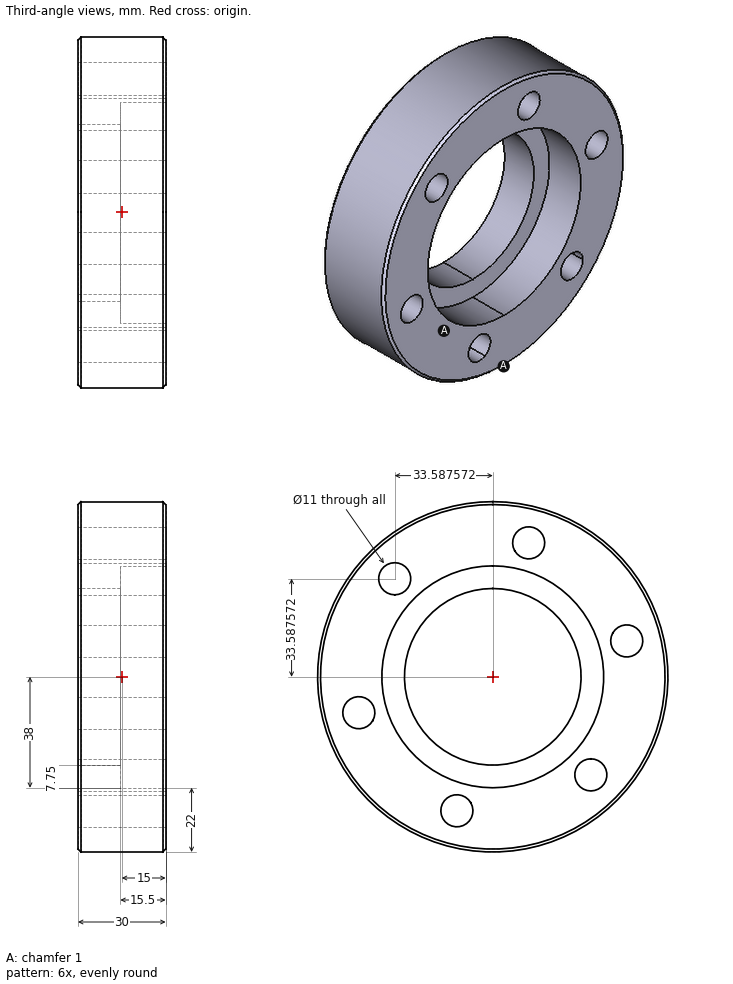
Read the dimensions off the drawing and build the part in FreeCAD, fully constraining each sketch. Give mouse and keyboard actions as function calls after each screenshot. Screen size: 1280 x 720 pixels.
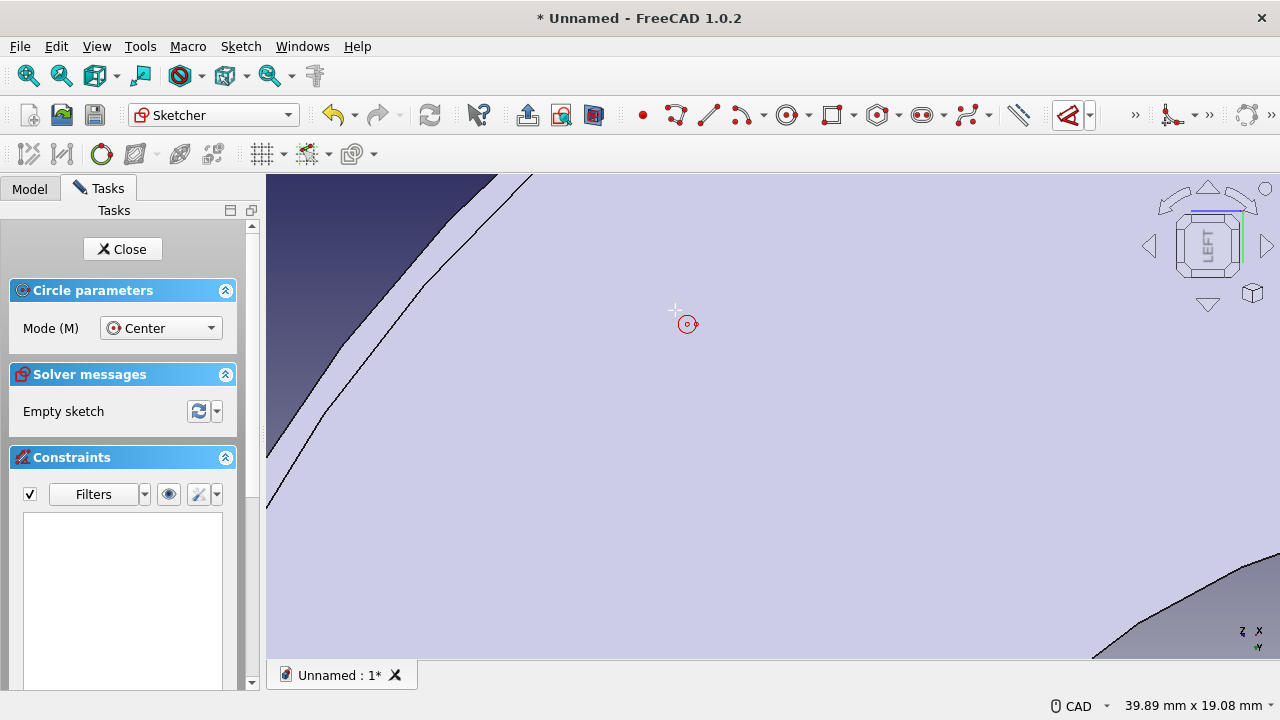
click(703, 415)
move(801, 316)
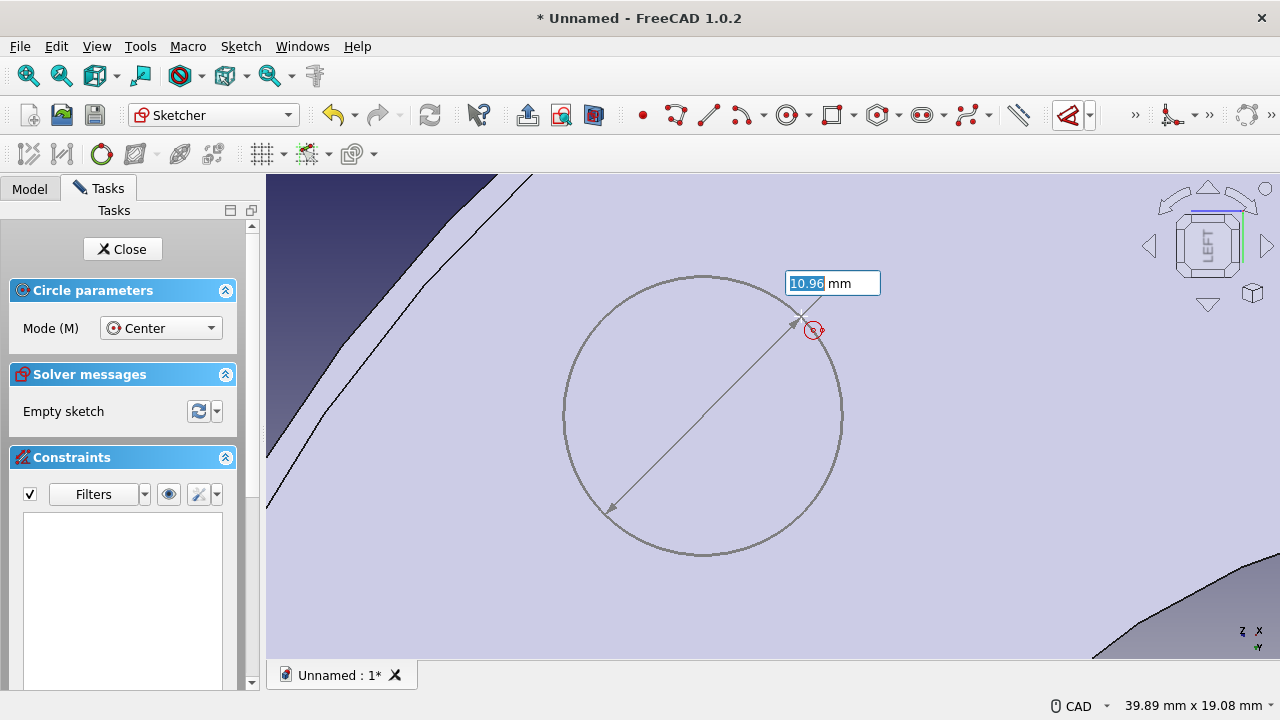
text(11)
key(Return)
key(Escape)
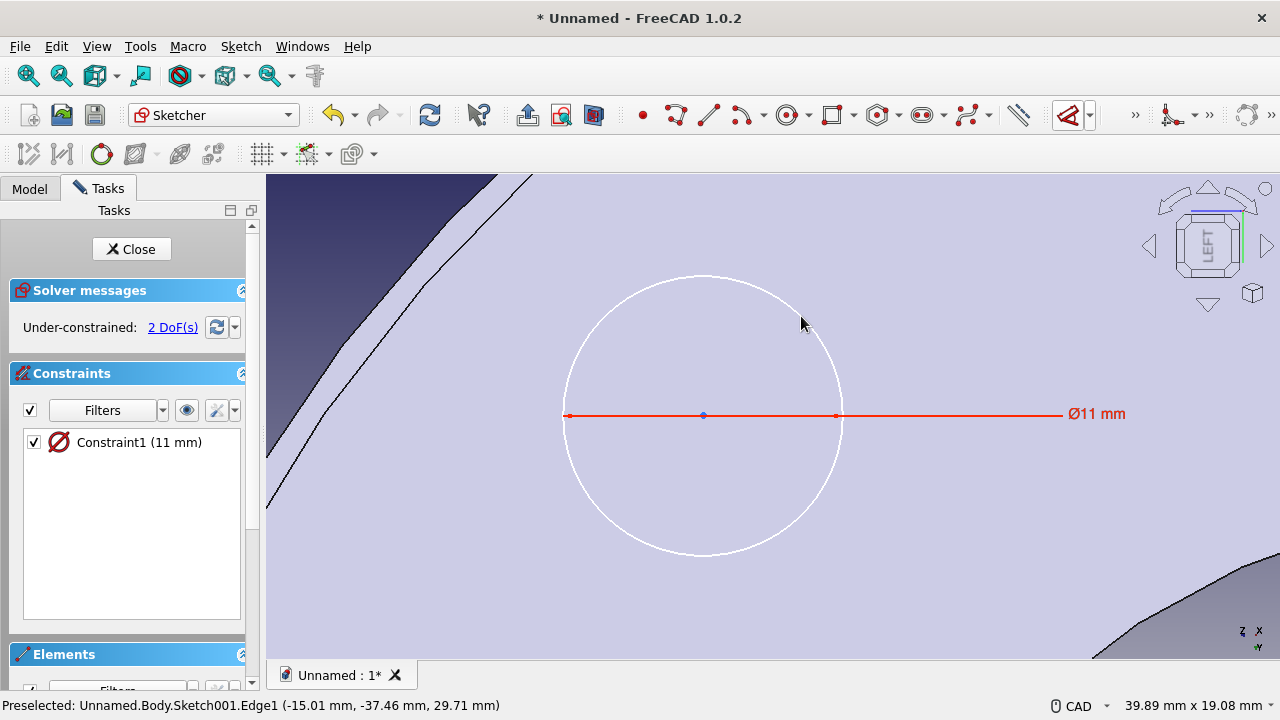
click(703, 416)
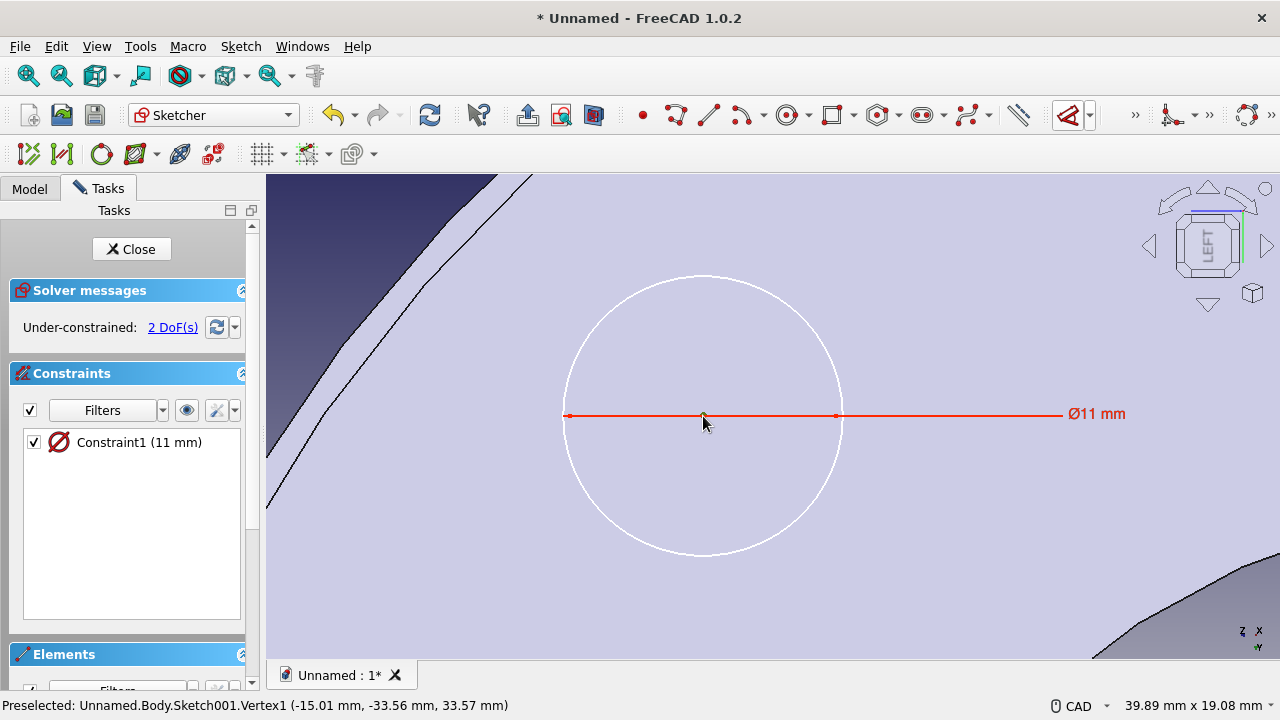
key(l)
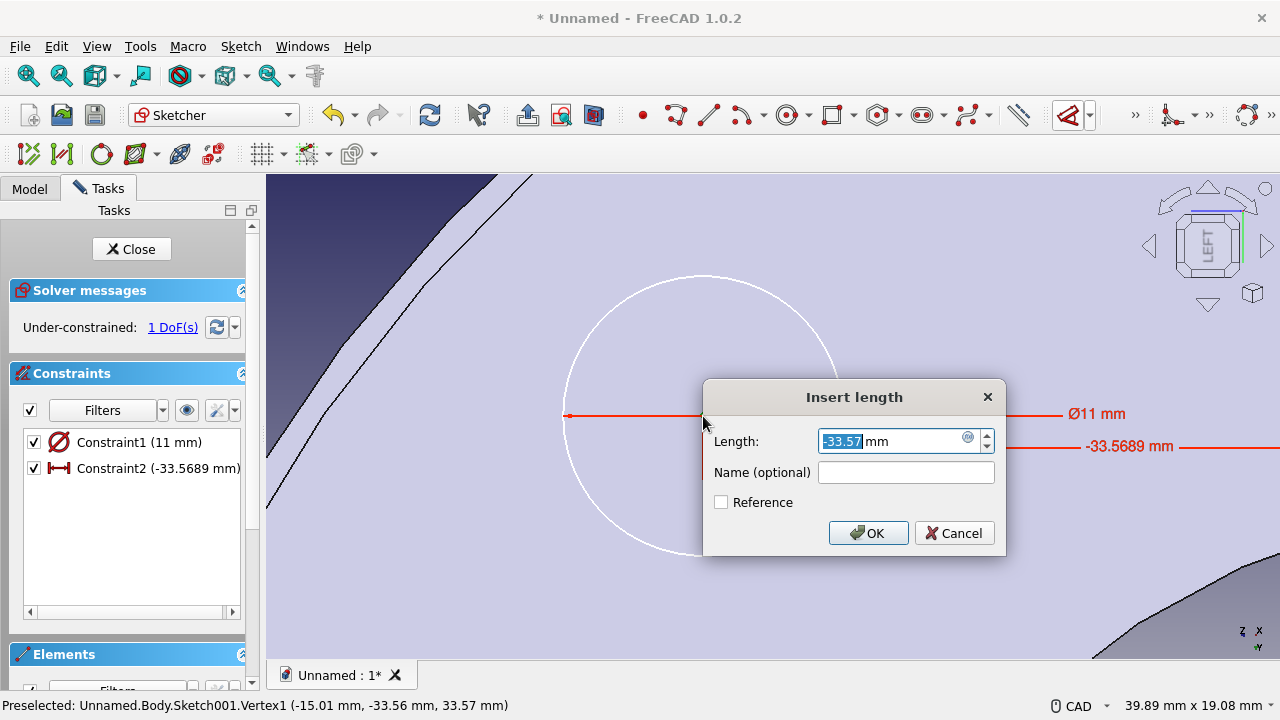
text(-33.587572)
key(Return)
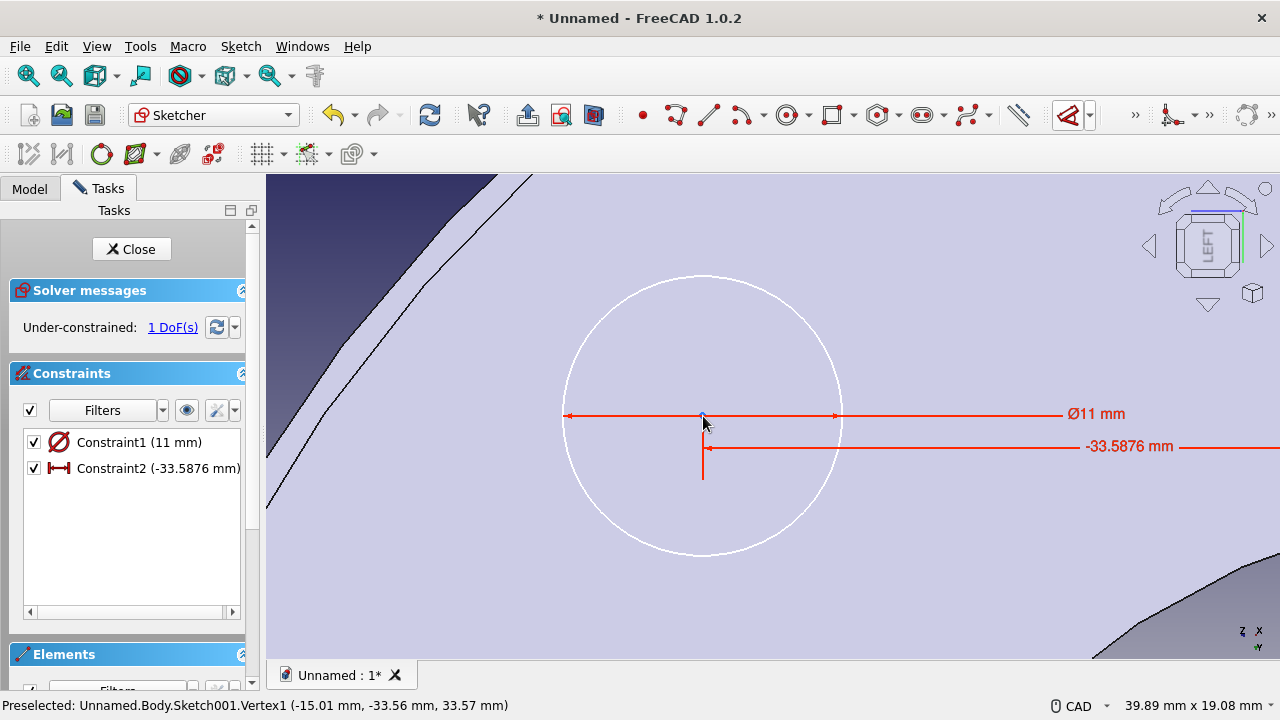
click(703, 416)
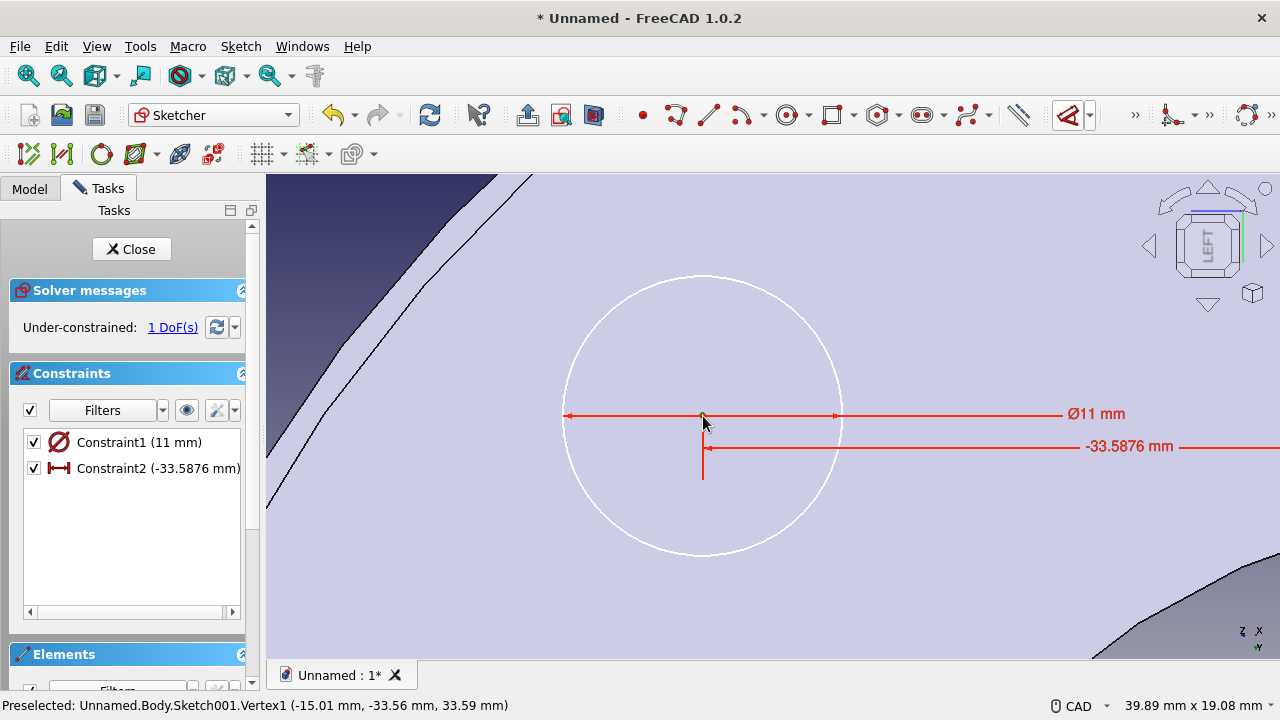
key(i)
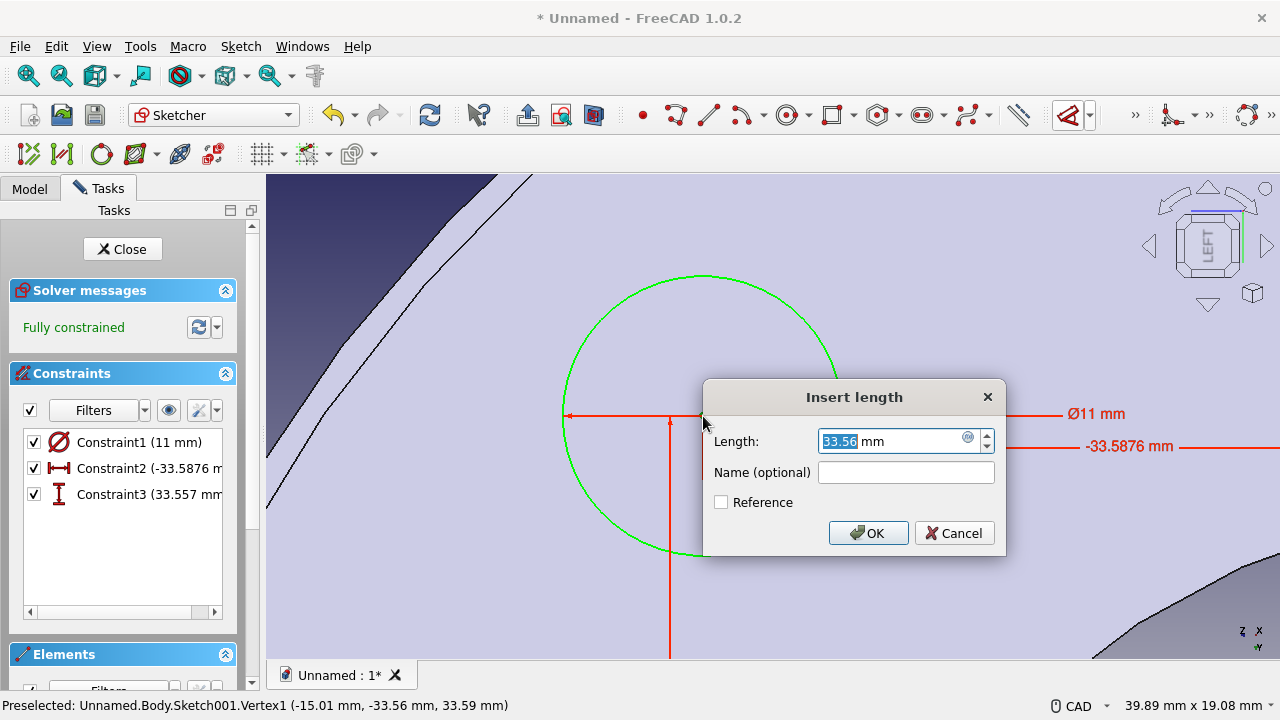
text(33.587572)
key(Return)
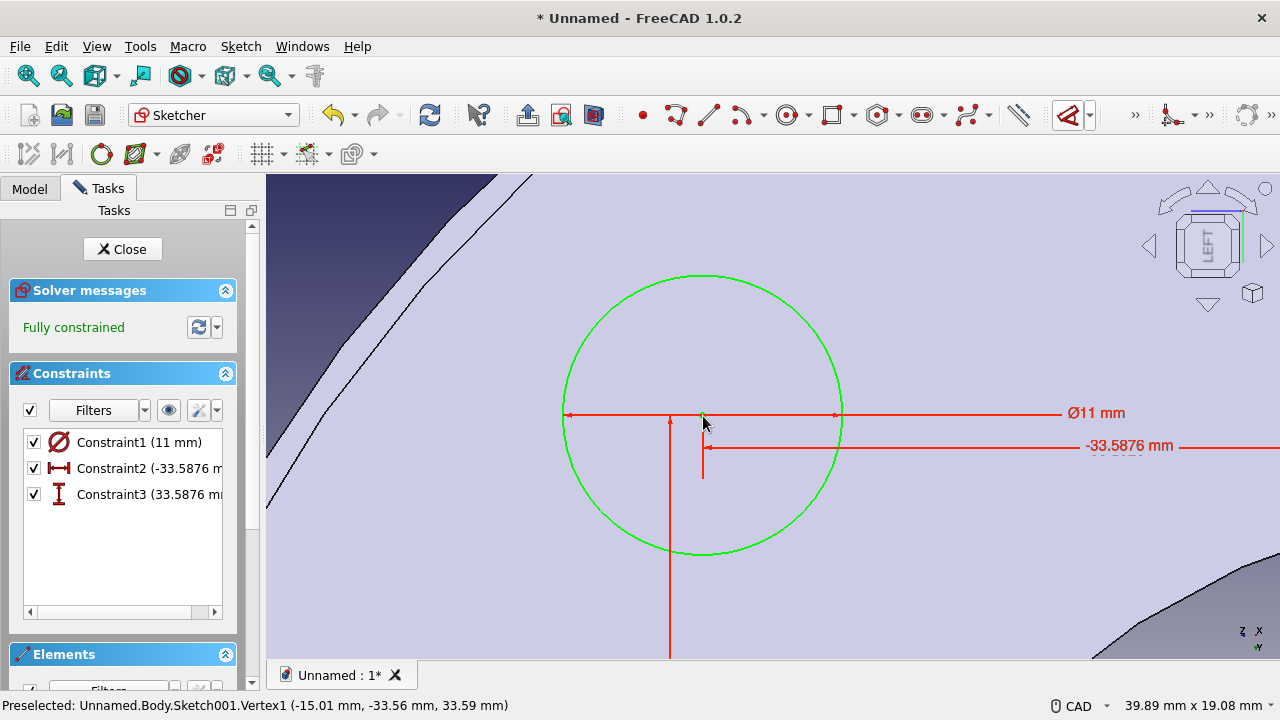
click(123, 249)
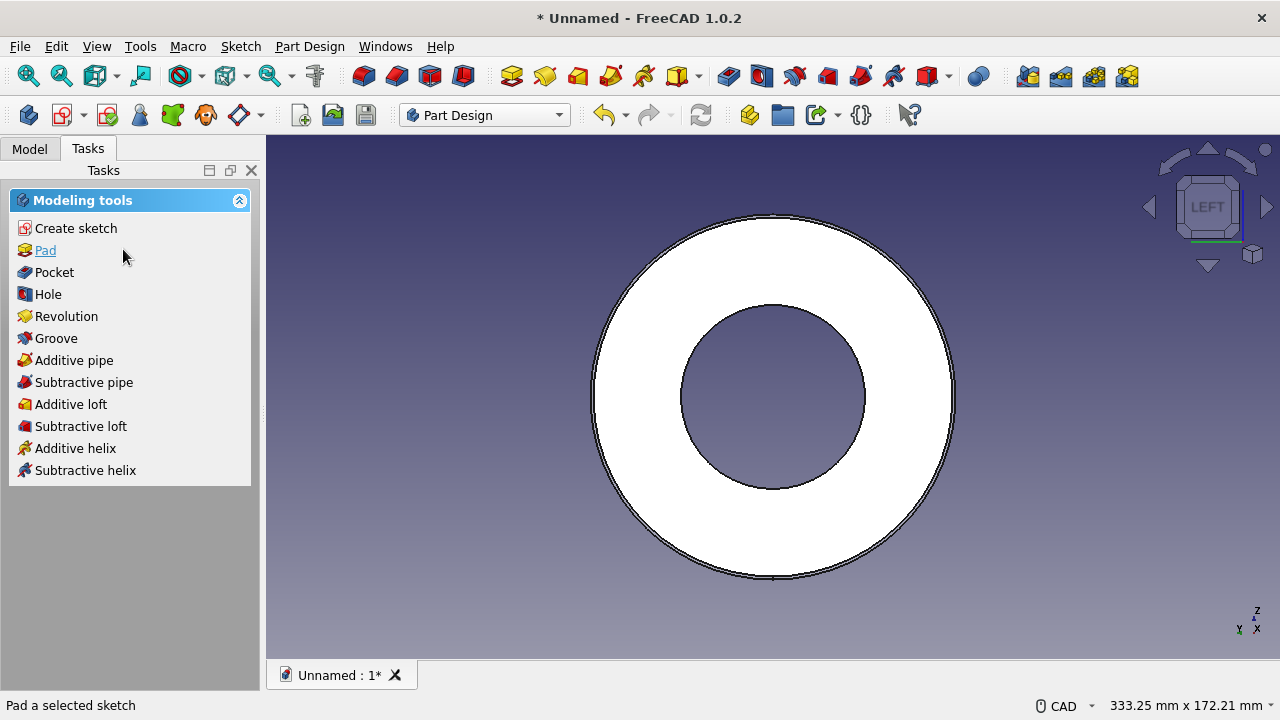
click(762, 76)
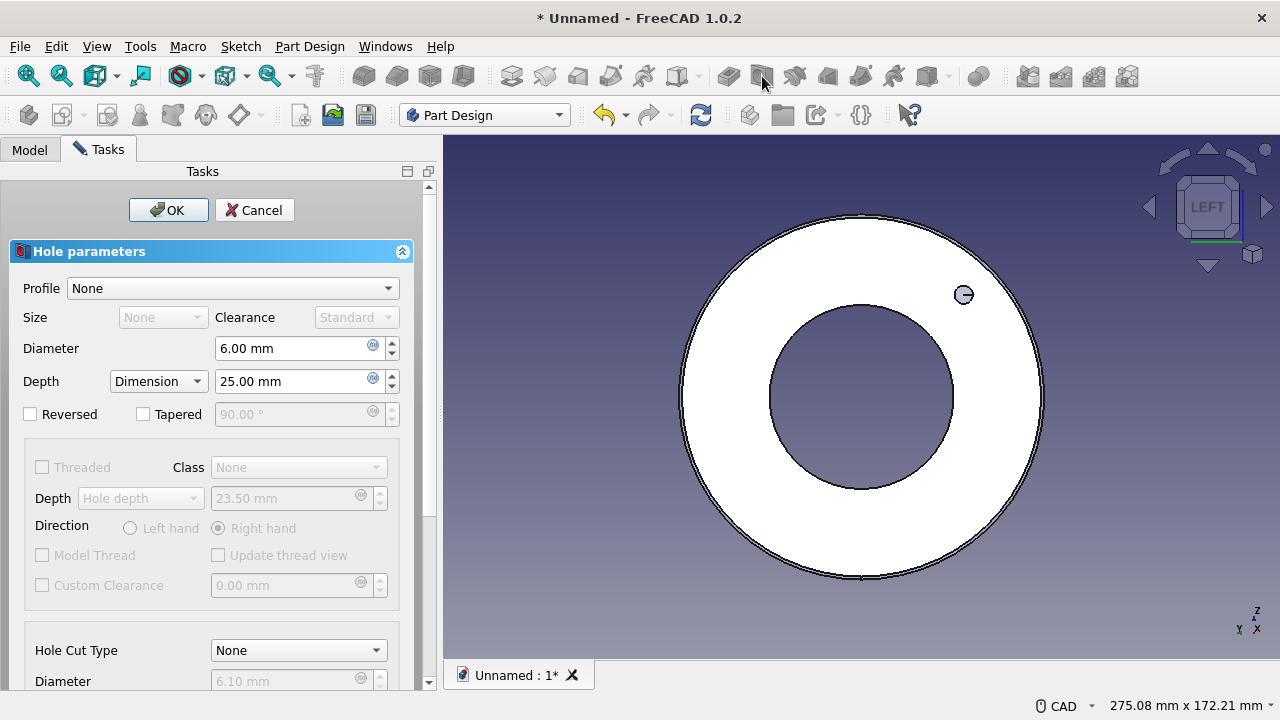
triple_click(300, 348)